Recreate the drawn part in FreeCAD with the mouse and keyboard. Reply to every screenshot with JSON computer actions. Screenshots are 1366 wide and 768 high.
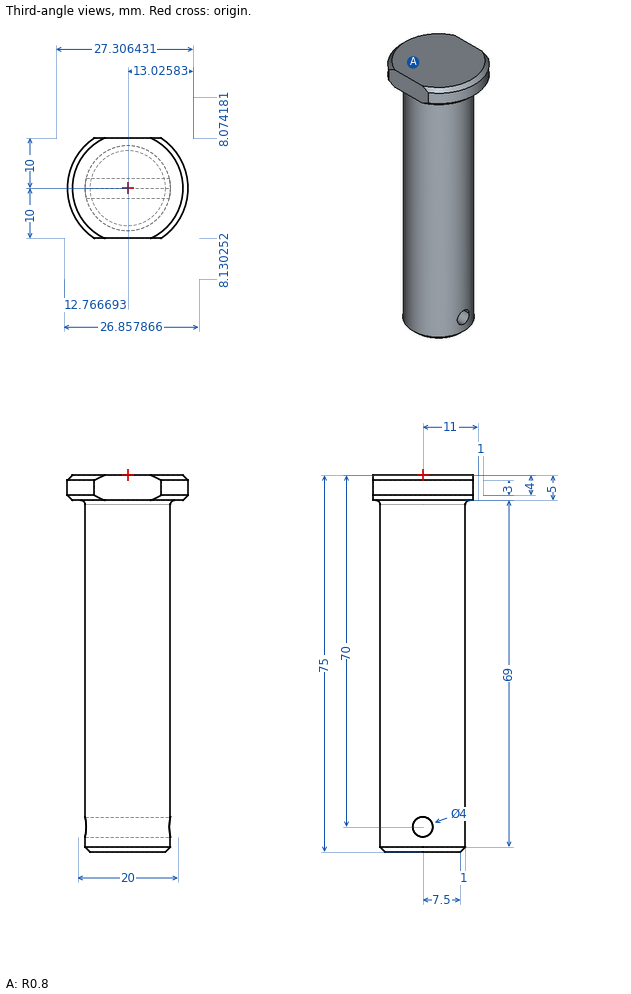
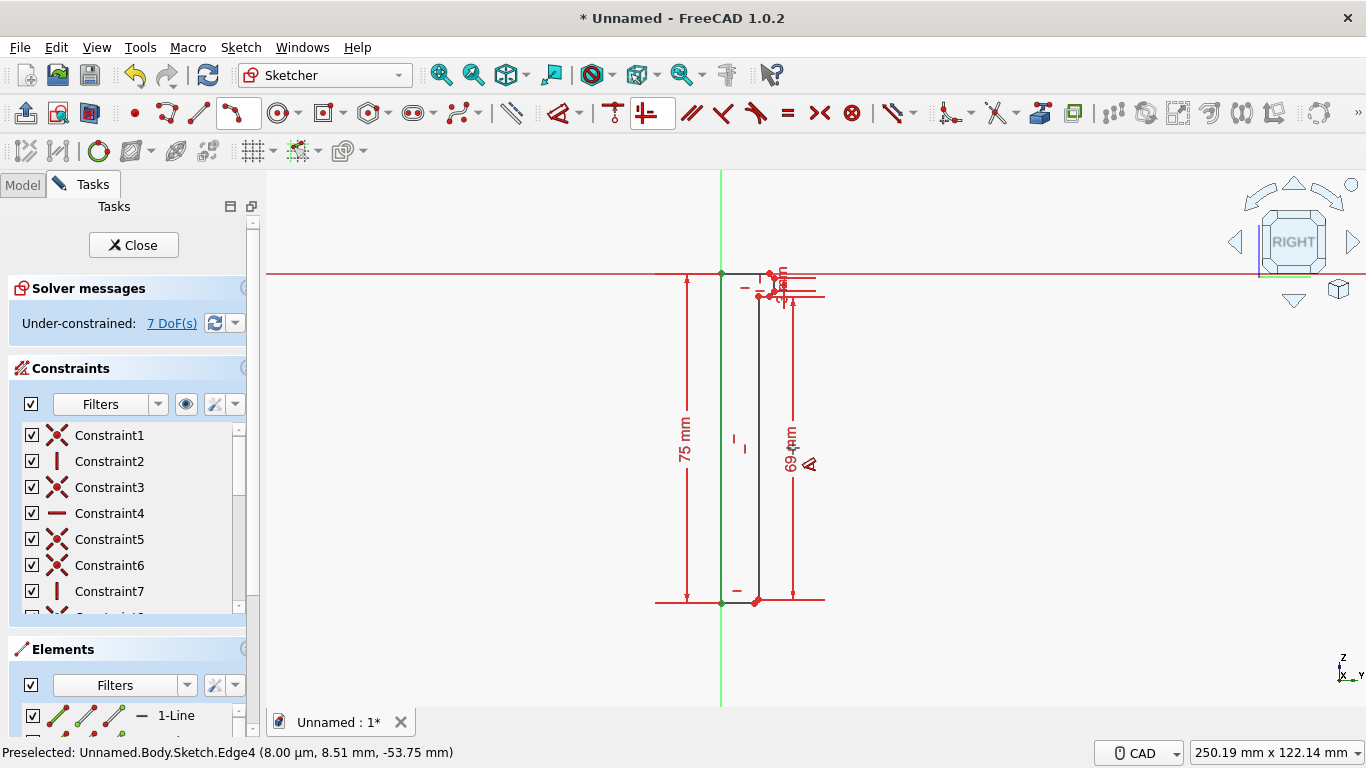
{"action": "left_click", "coordinate": [755, 274]}
{"action": "left_click", "coordinate": [746, 240]}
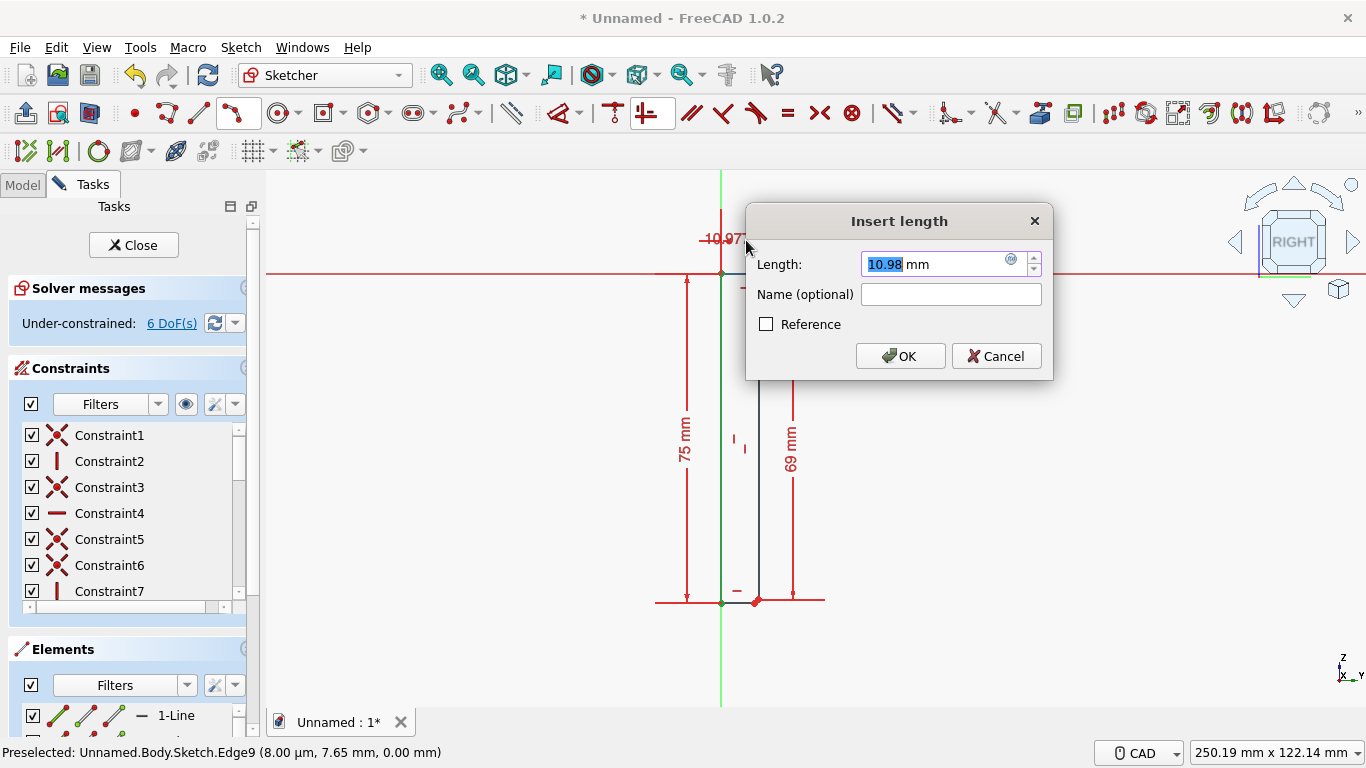
{"action": "type", "text": "11"}
{"action": "key", "text": "Return"}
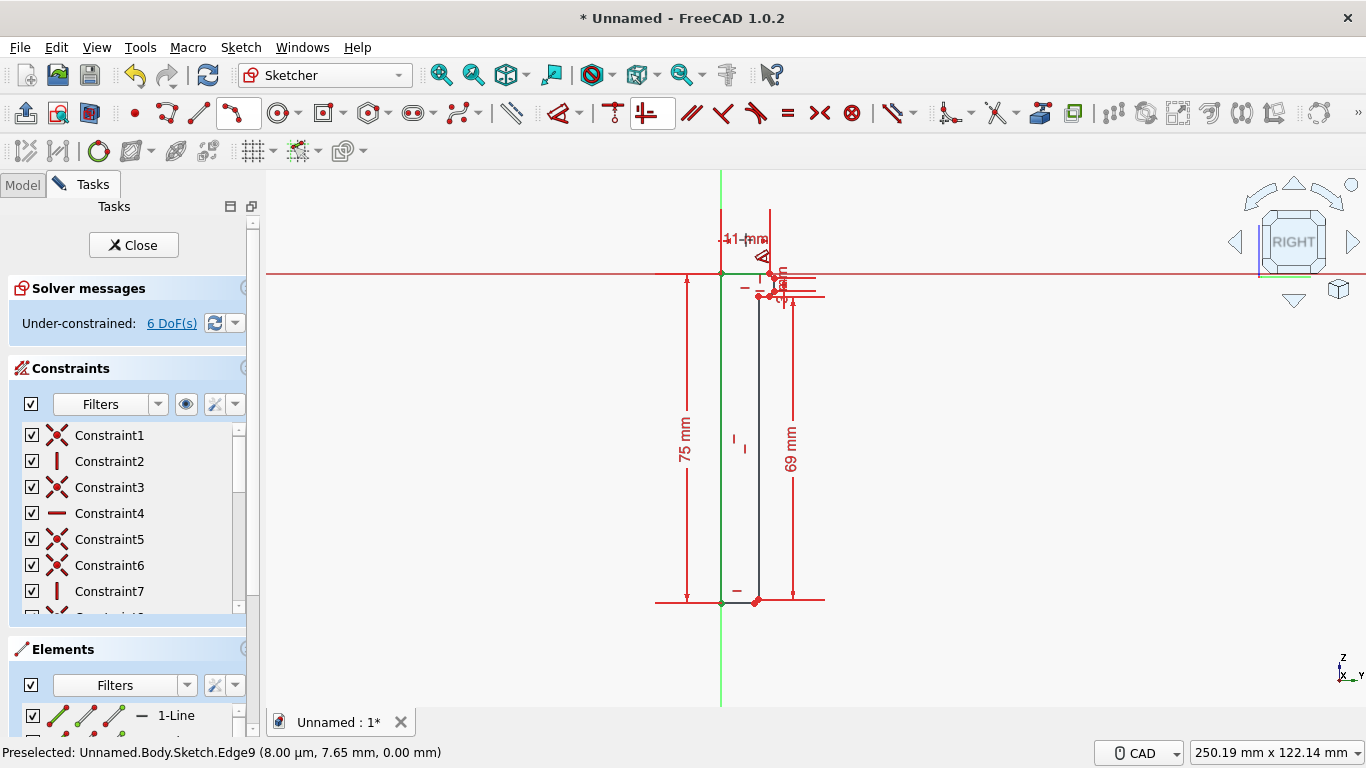
{"action": "scroll", "coordinate": [759, 297], "scroll_direction": "up", "scroll_amount": 3}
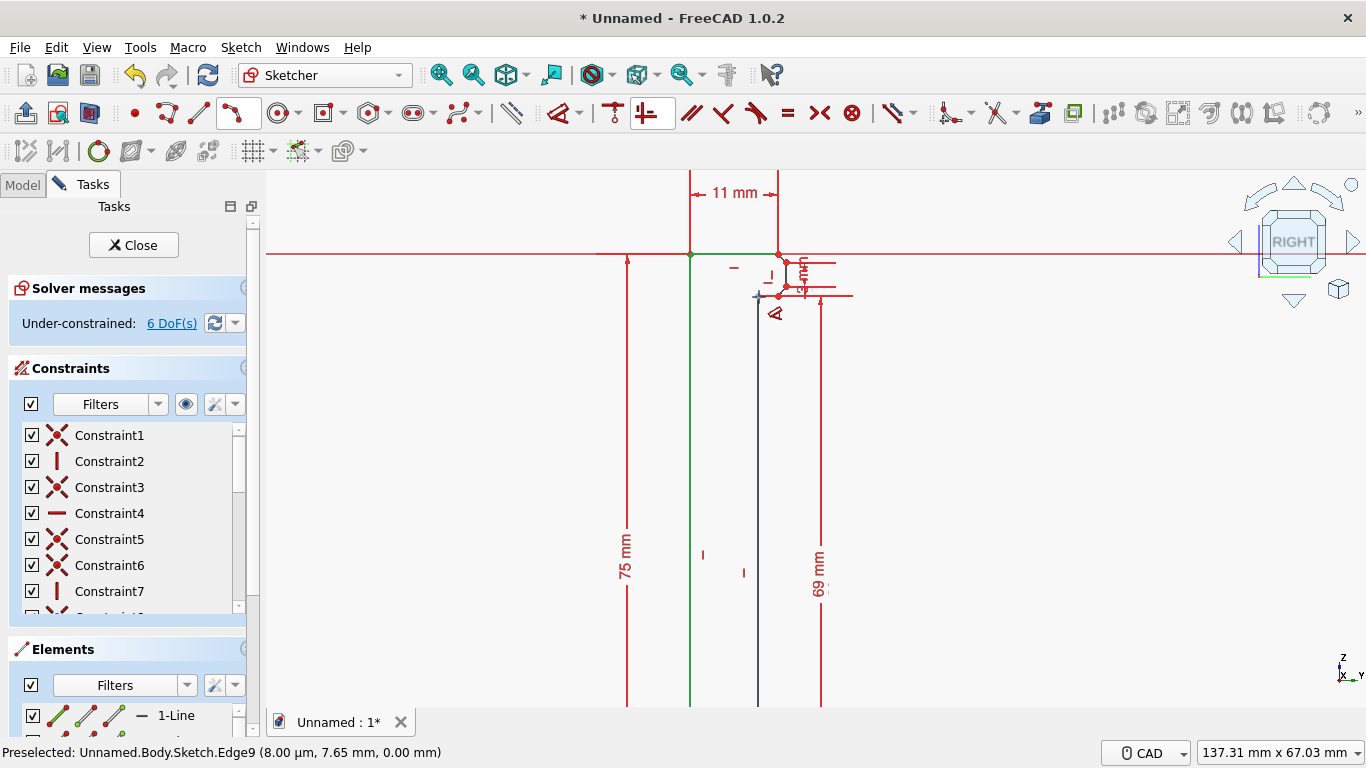
{"action": "left_click", "coordinate": [758, 296]}
{"action": "left_click", "coordinate": [656, 275]}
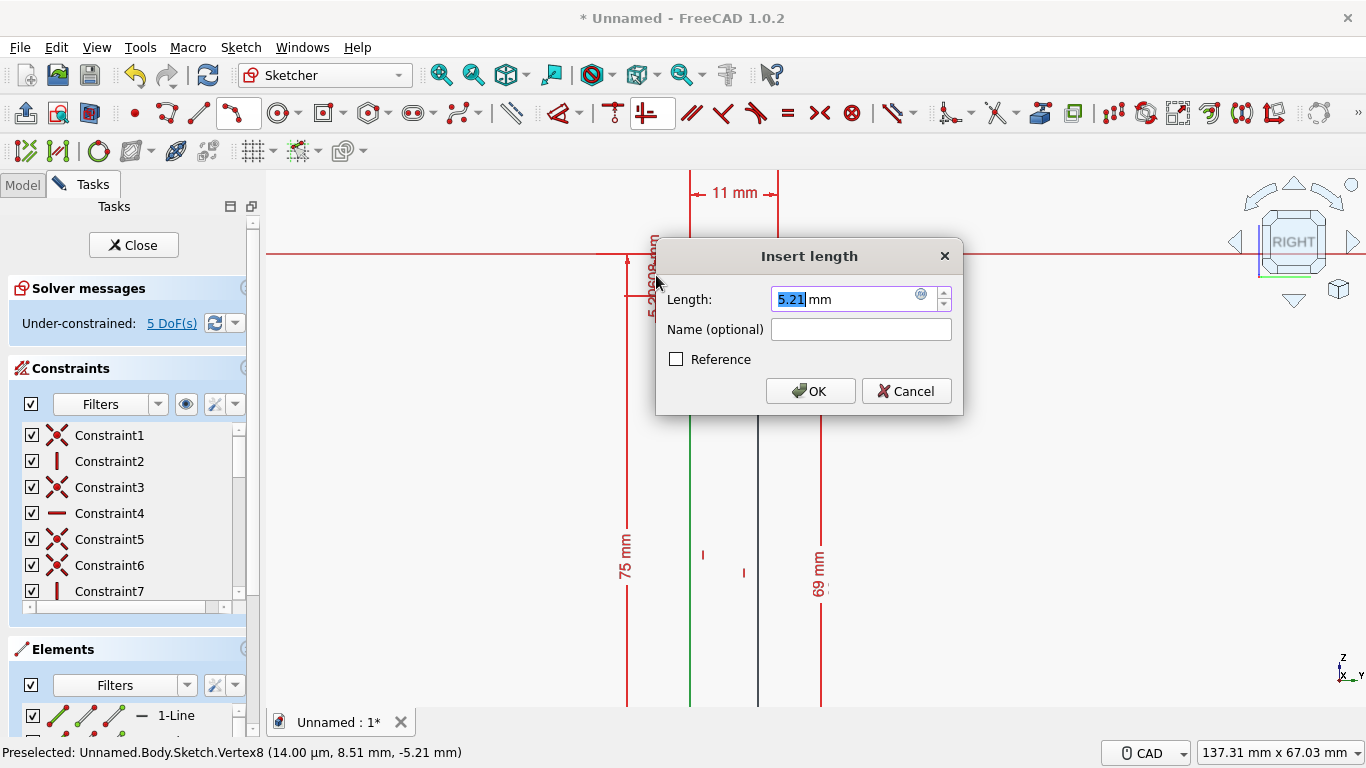
{"action": "type", "text": "5"}
{"action": "key", "text": "Return"}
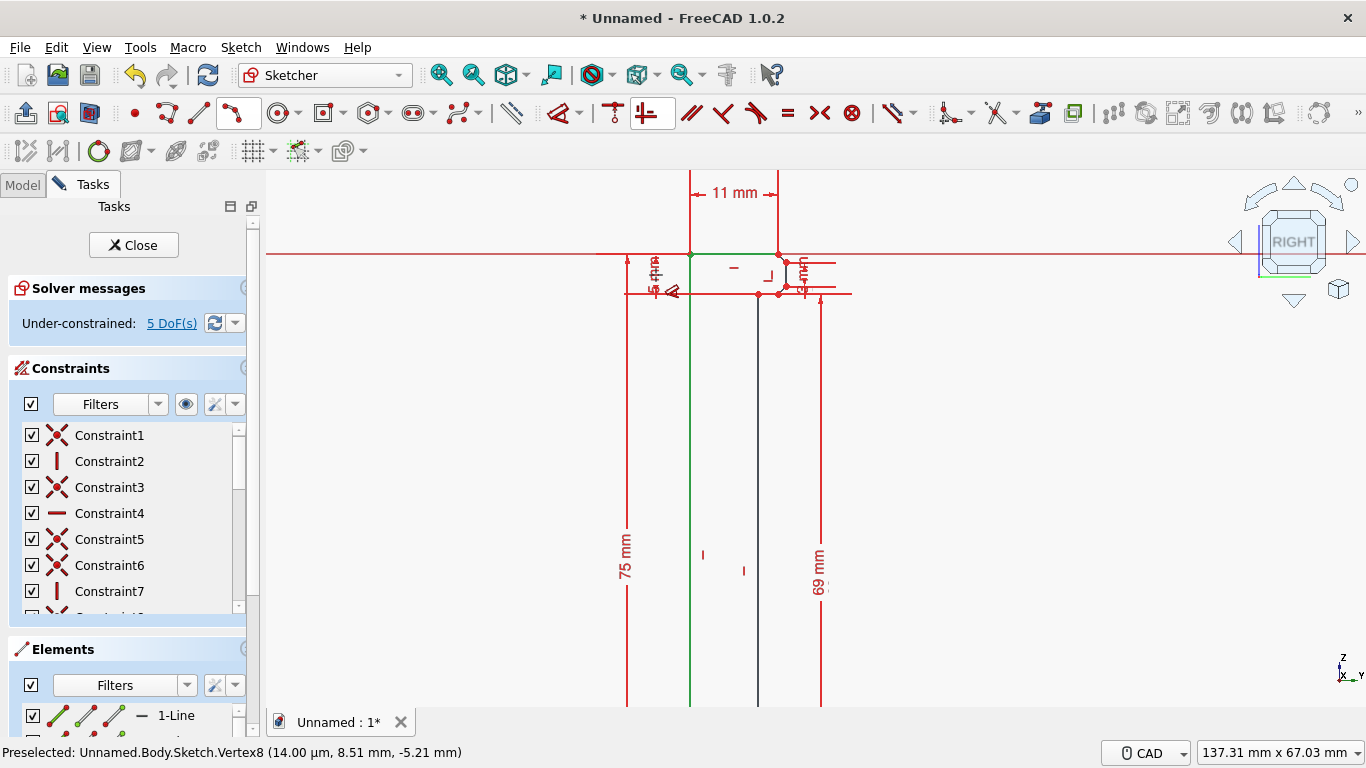
{"action": "scroll", "coordinate": [786, 287], "scroll_direction": "up", "scroll_amount": 2}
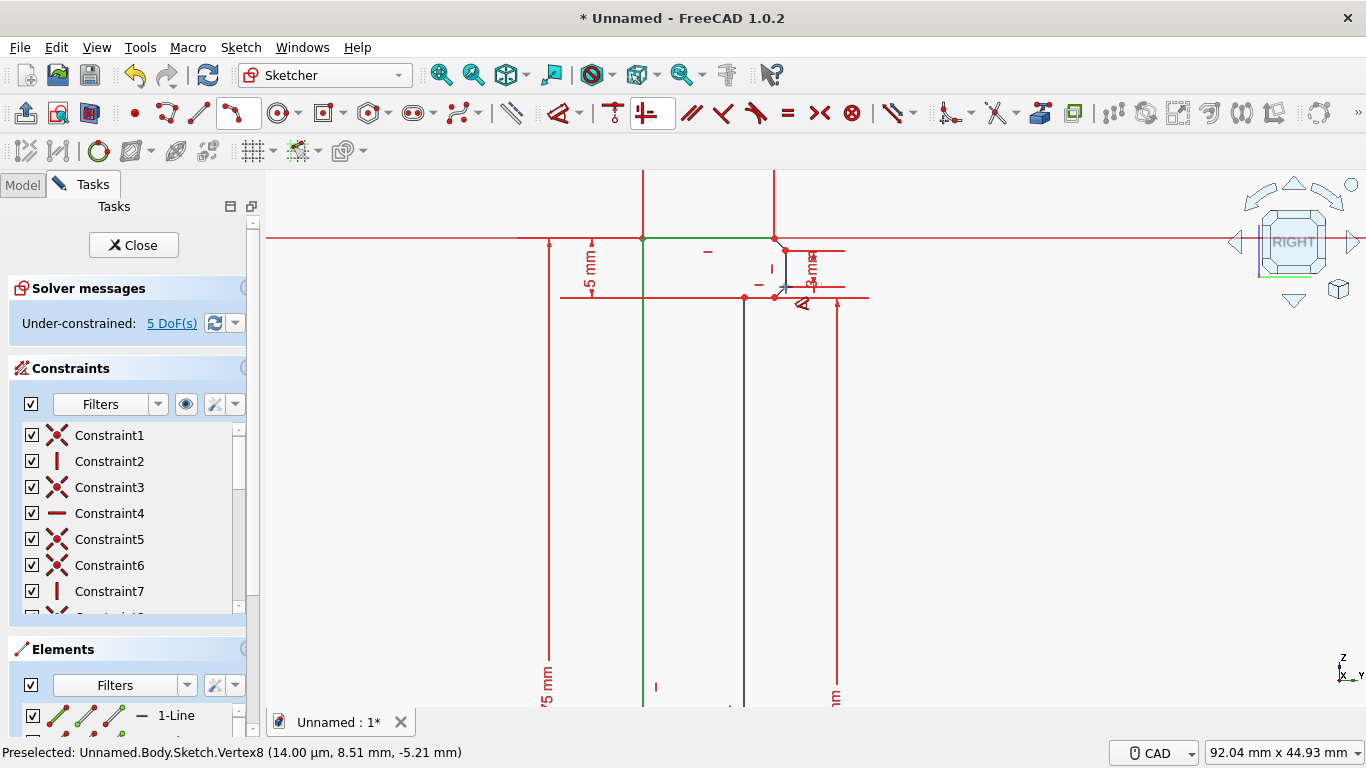
{"action": "left_click", "coordinate": [786, 287]}
{"action": "left_click", "coordinate": [892, 262]}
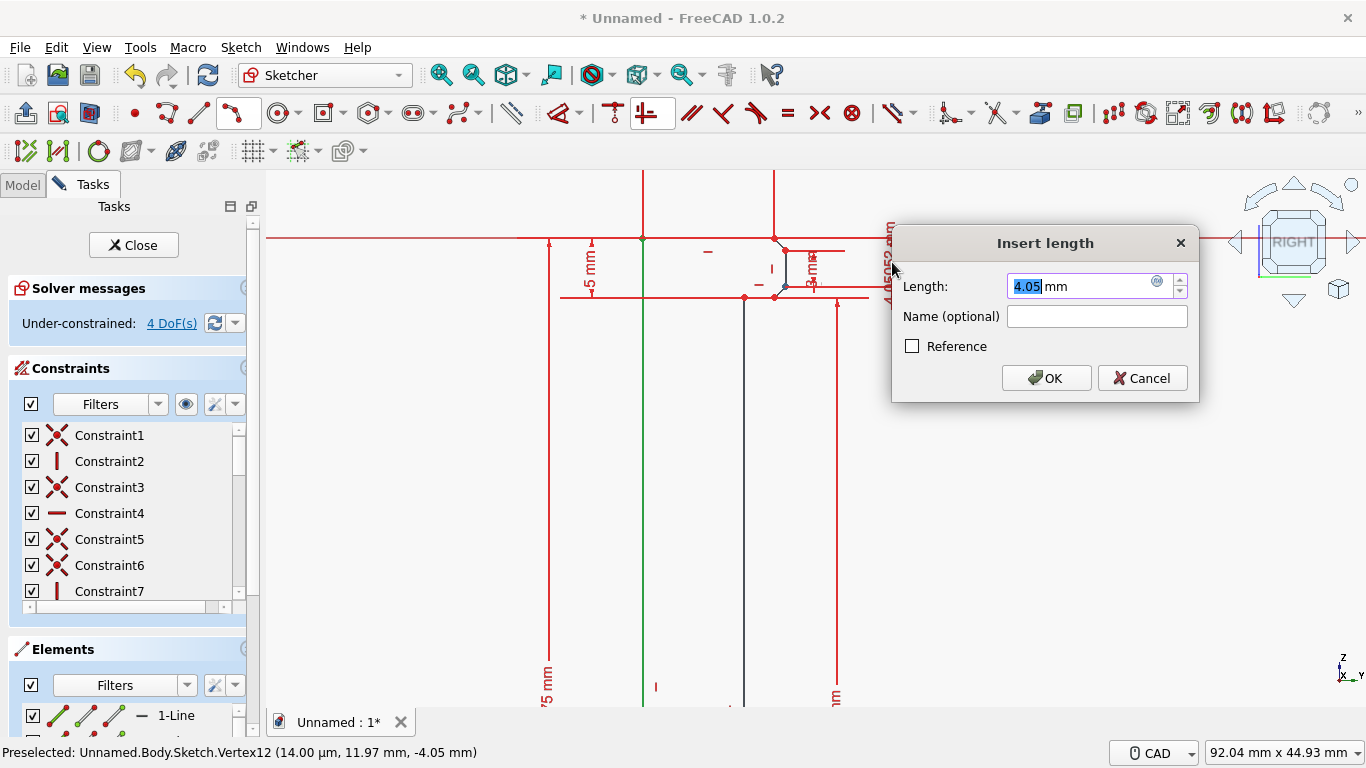
{"action": "type", "text": "4"}
{"action": "key", "text": "Return"}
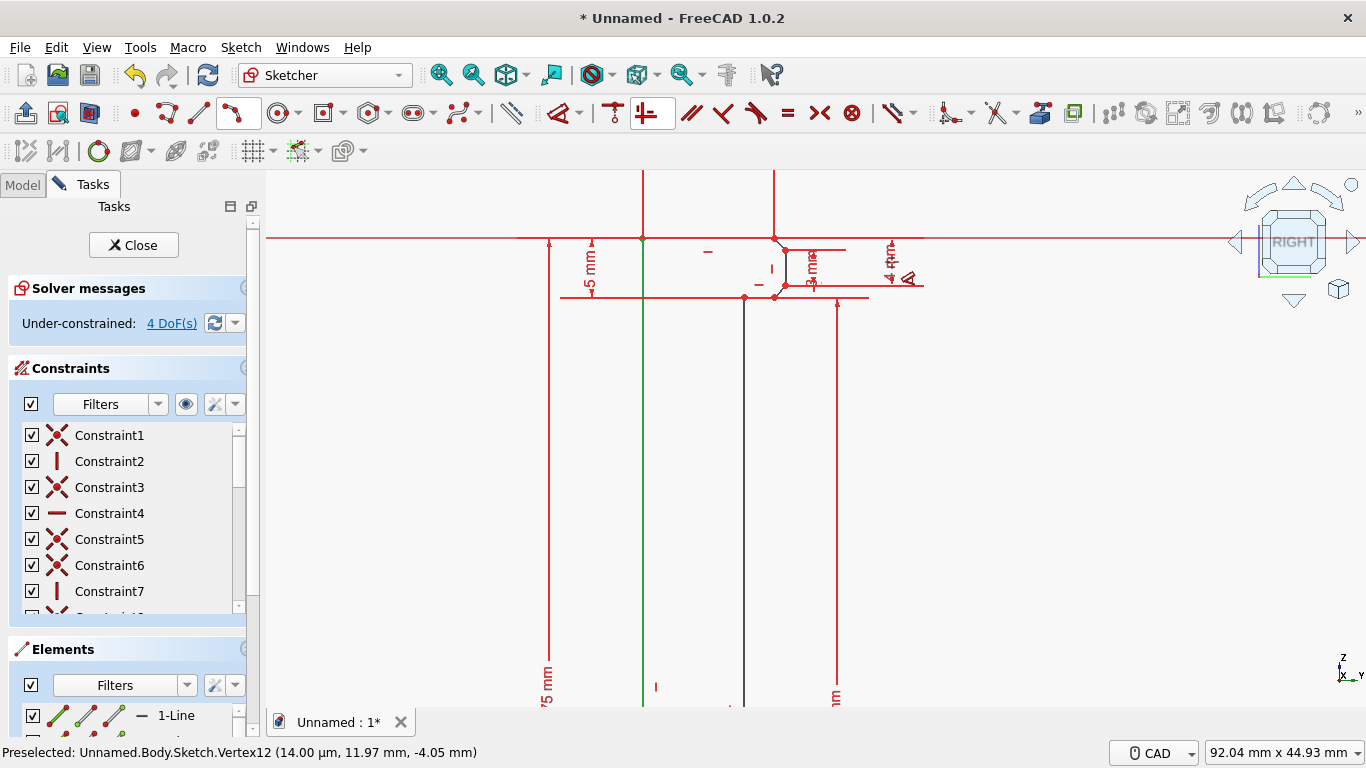
{"action": "scroll", "coordinate": [767, 294], "scroll_direction": "down", "scroll_amount": 5}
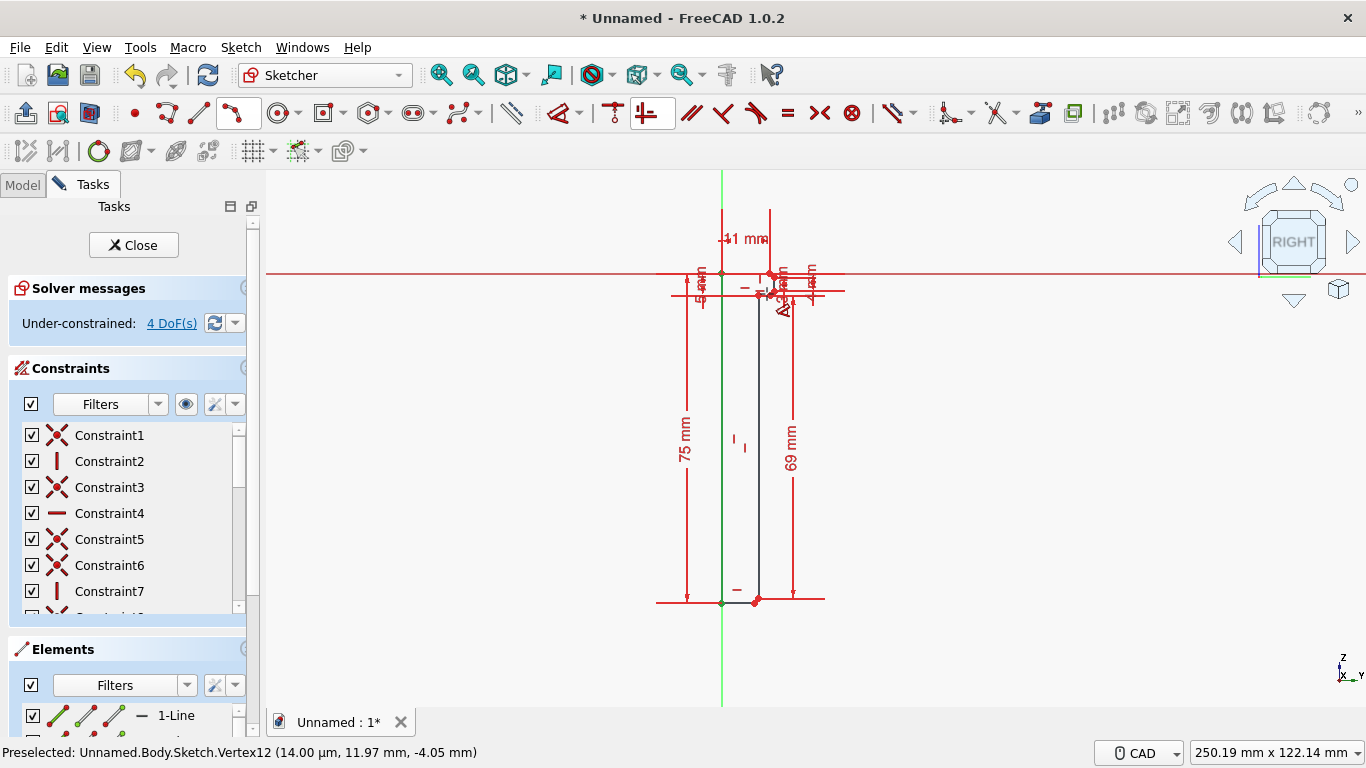
{"action": "scroll", "coordinate": [757, 601], "scroll_direction": "up", "scroll_amount": 12}